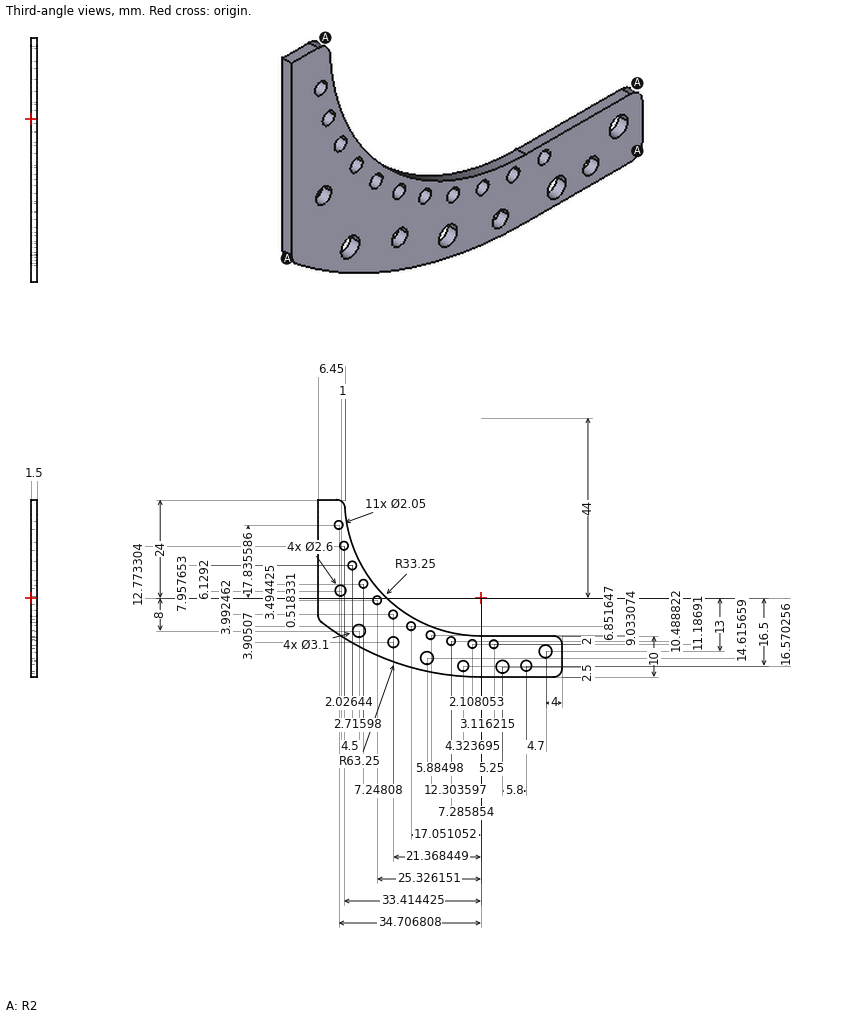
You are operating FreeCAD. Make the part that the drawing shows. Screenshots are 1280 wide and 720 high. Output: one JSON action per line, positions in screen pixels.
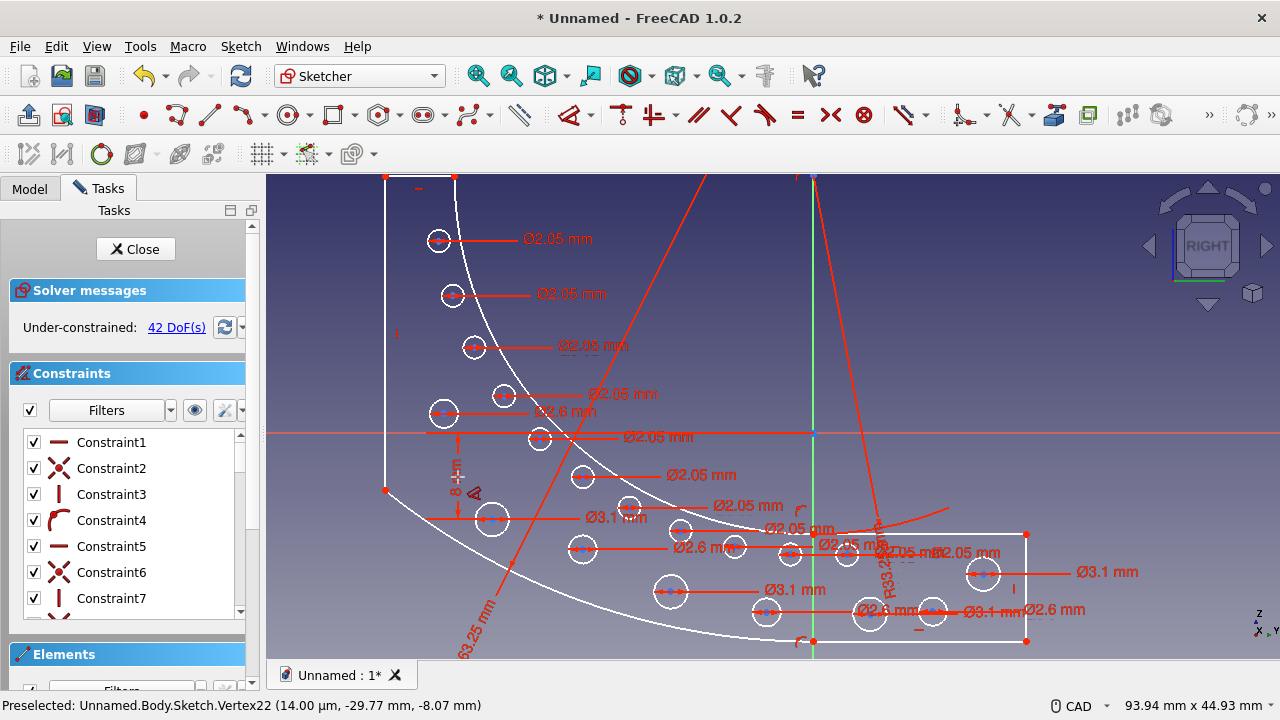
{"action": "left_click", "coordinate": [1026, 609]}
{"action": "left_click", "coordinate": [1060, 583]}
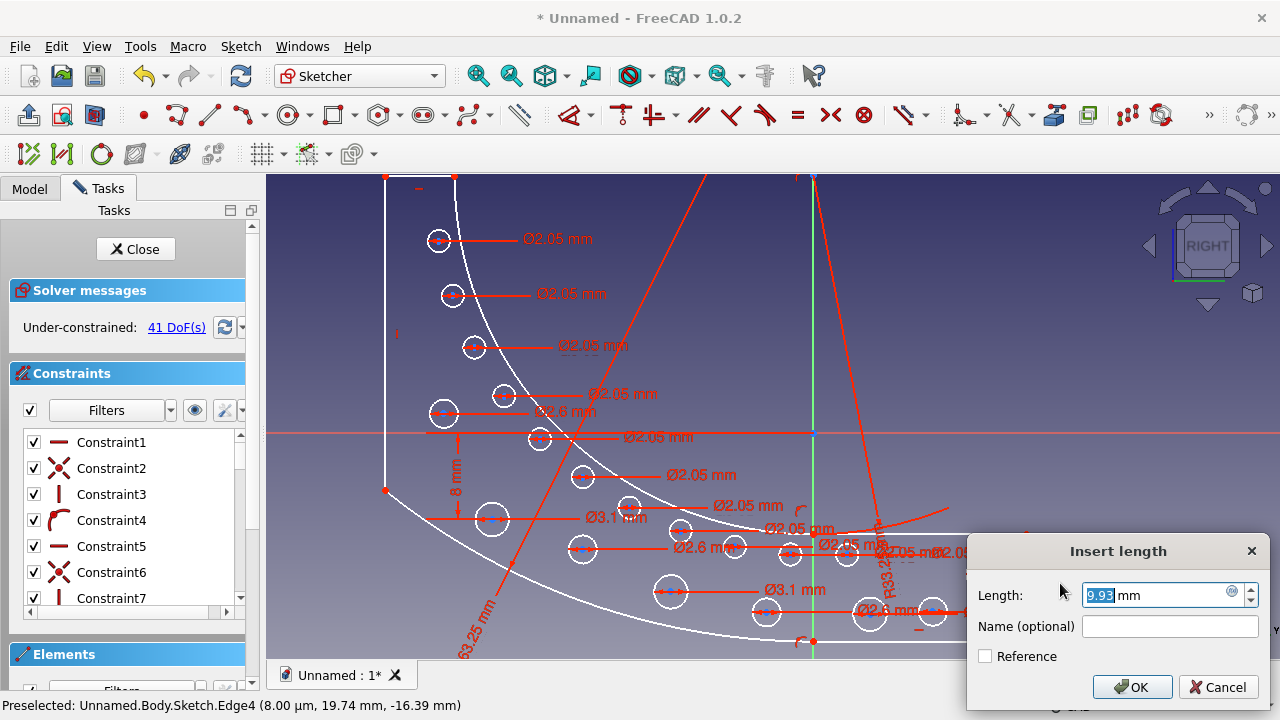
{"action": "type", "text": "10"}
{"action": "key", "text": "Return"}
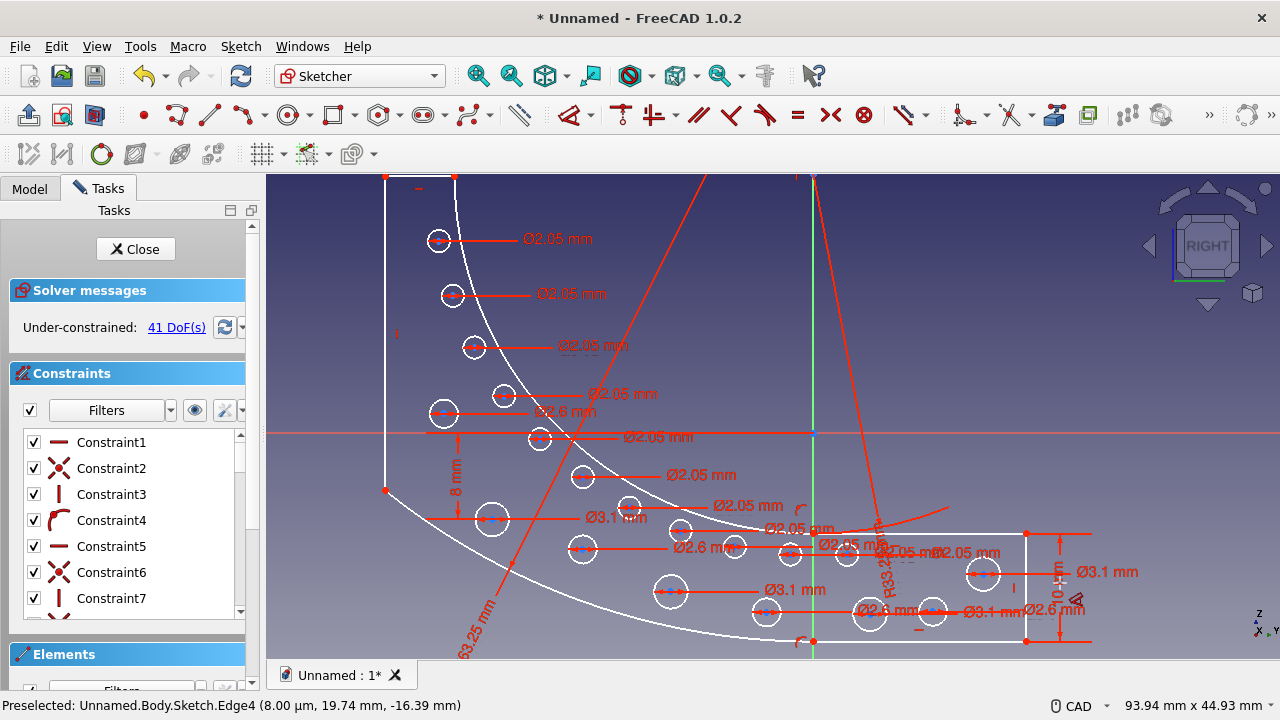
{"action": "left_click", "coordinate": [983, 574]}
{"action": "left_click", "coordinate": [1017, 504]}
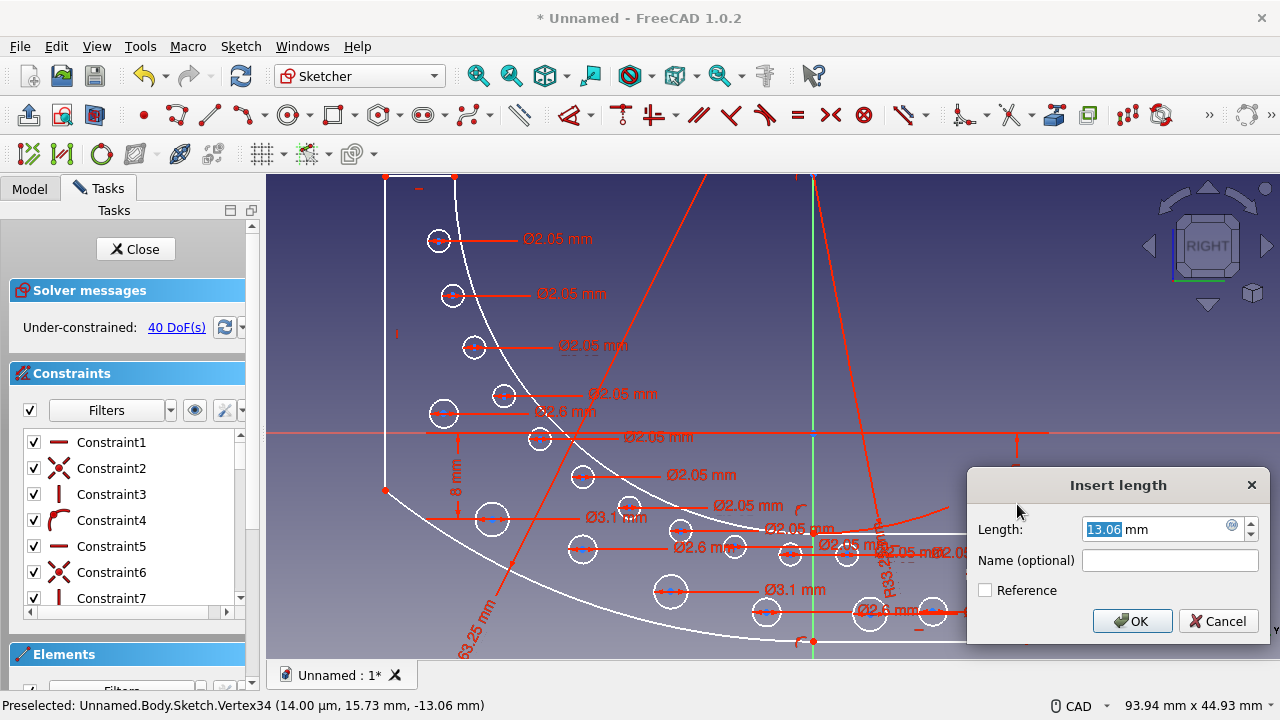
{"action": "type", "text": "13"}
{"action": "key", "text": "Return"}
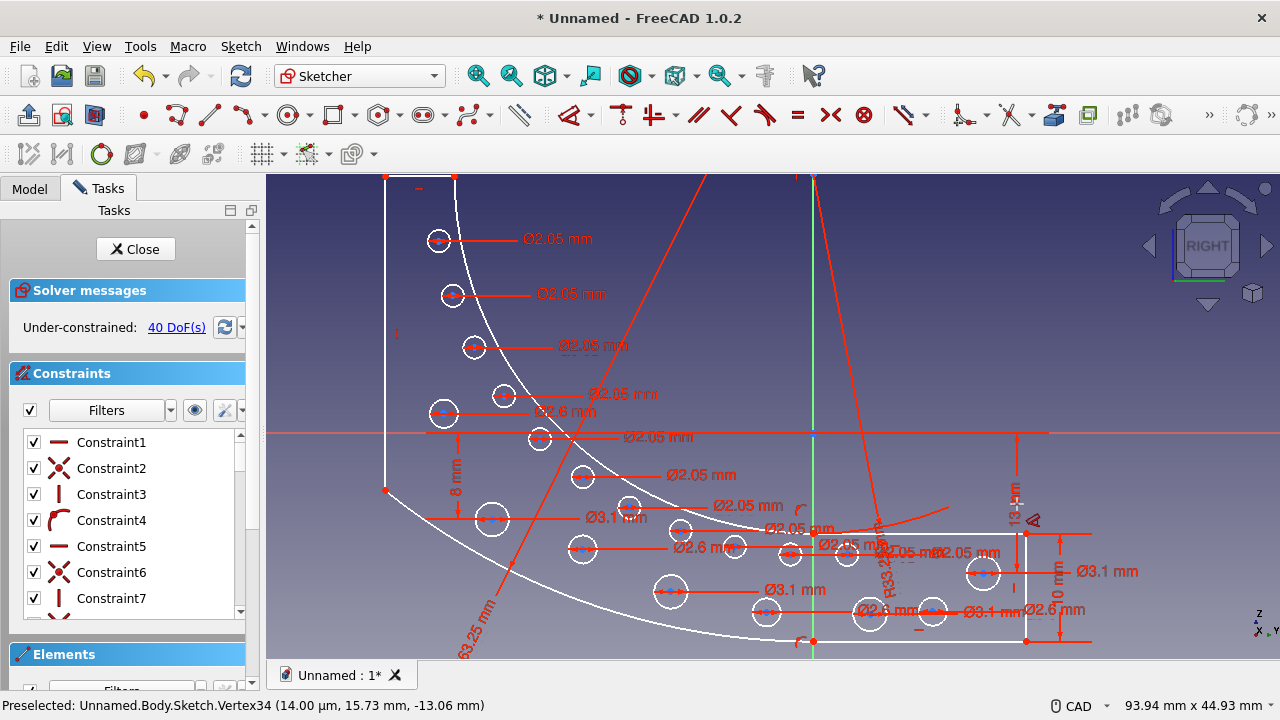
{"action": "scroll", "coordinate": [702, 435], "scroll_direction": "down", "scroll_amount": 2}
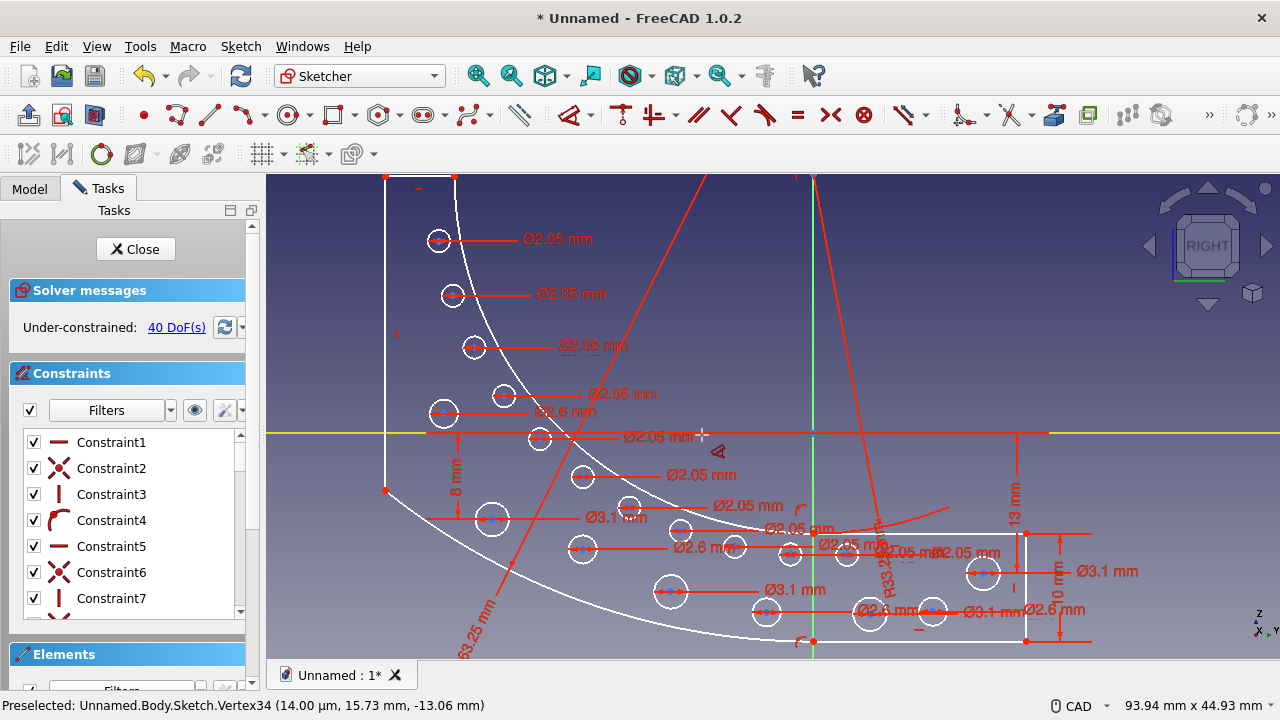
{"action": "scroll", "coordinate": [536, 262], "scroll_direction": "up", "scroll_amount": 9}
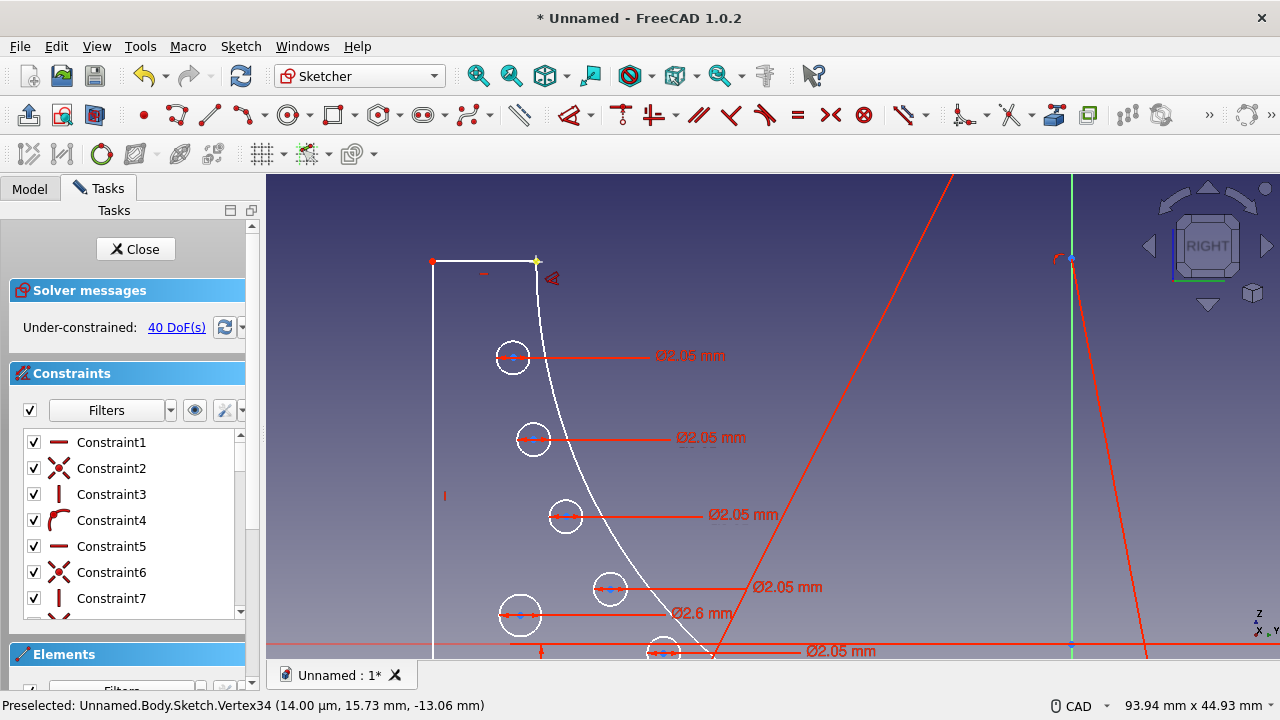
{"action": "left_click", "coordinate": [536, 259]}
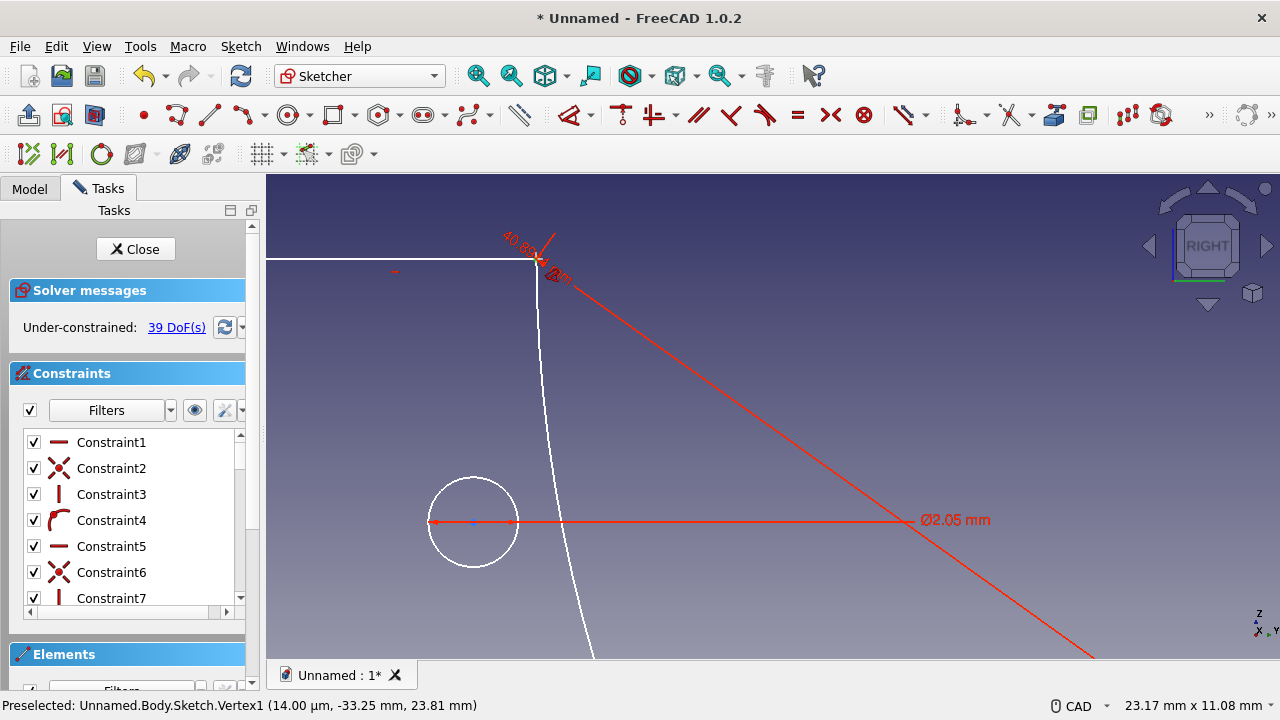
{"action": "scroll", "coordinate": [536, 262], "scroll_direction": "down", "scroll_amount": 9}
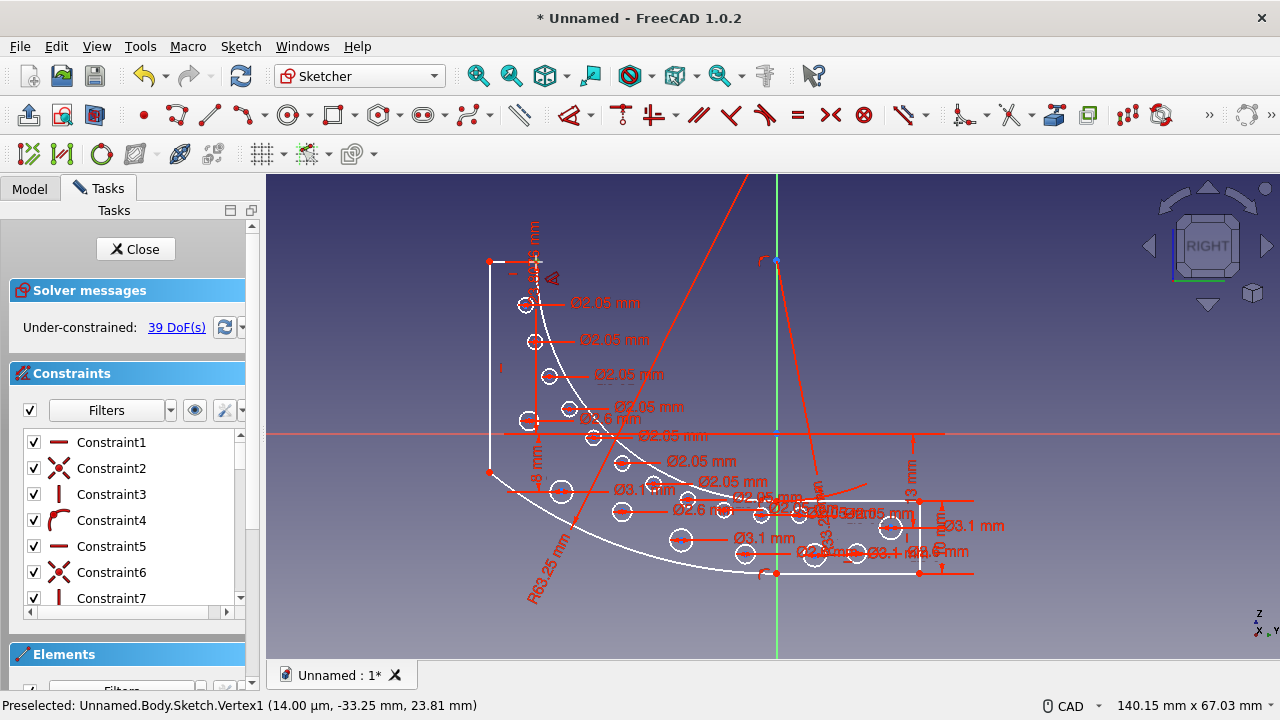
{"action": "scroll", "coordinate": [529, 421], "scroll_direction": "up", "scroll_amount": 9}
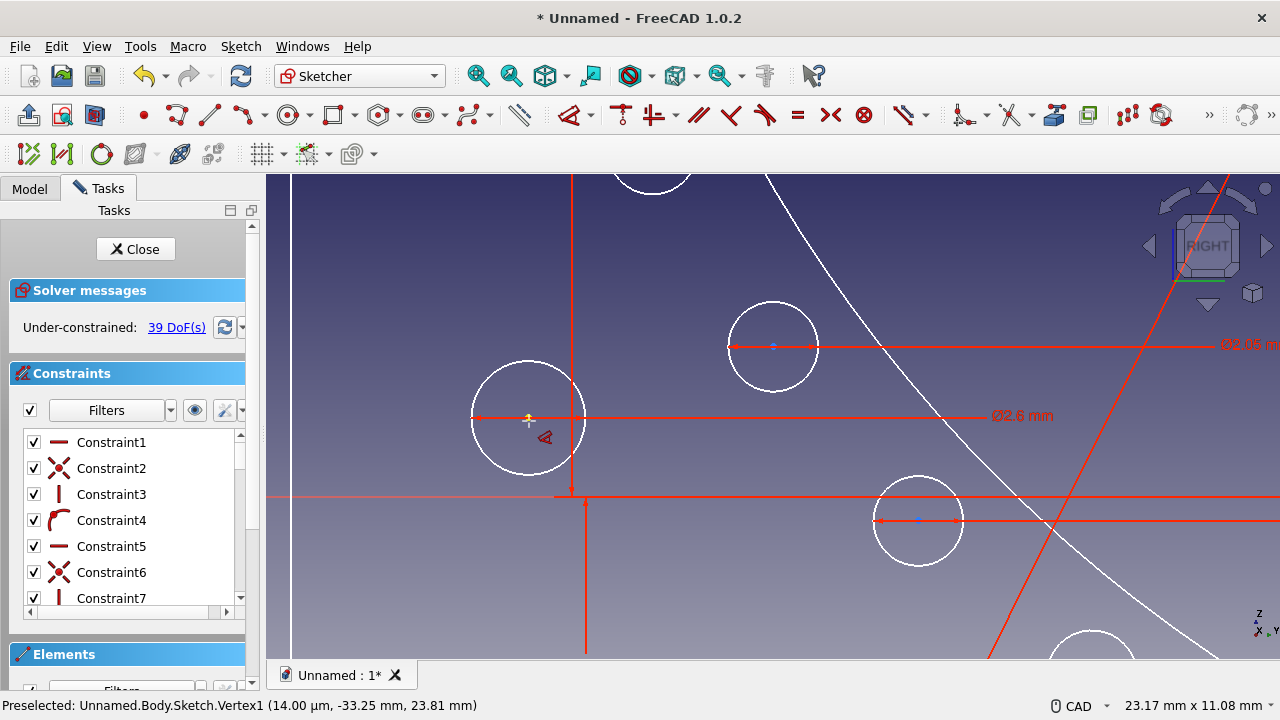
{"action": "left_click", "coordinate": [528, 418]}
{"action": "left_click", "coordinate": [550, 452]}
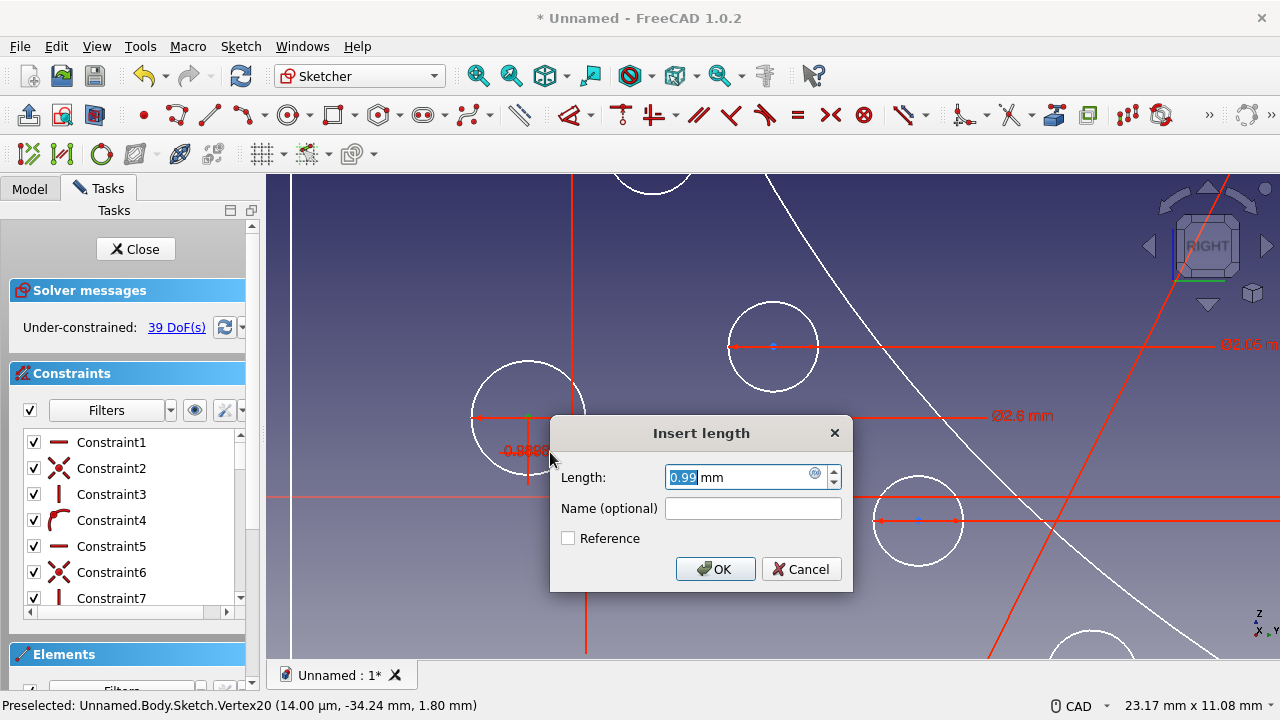
{"action": "type", "text": "1"}
{"action": "key", "text": "Return"}